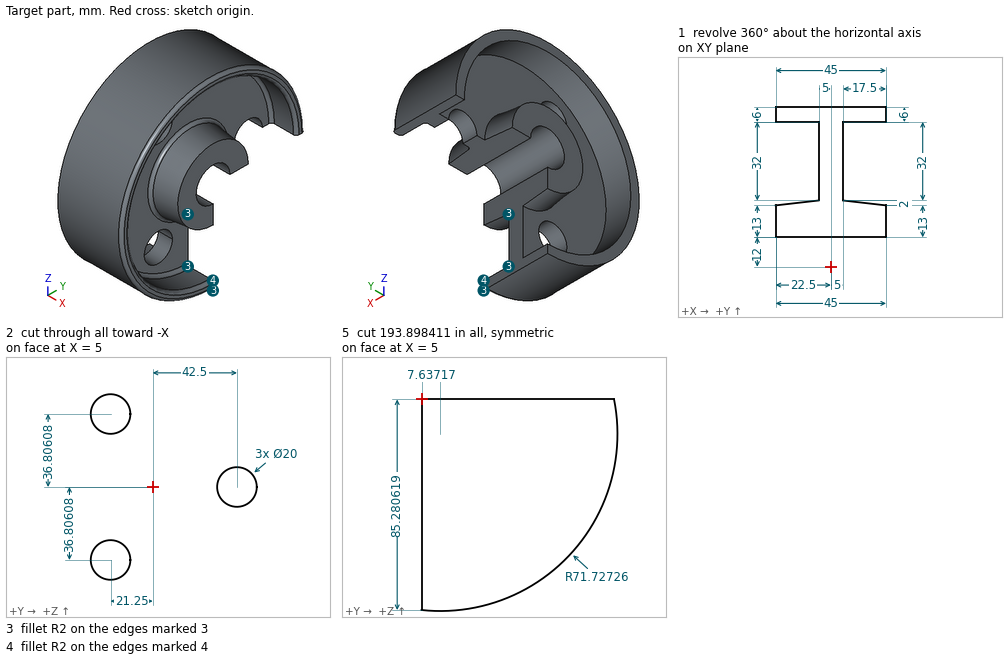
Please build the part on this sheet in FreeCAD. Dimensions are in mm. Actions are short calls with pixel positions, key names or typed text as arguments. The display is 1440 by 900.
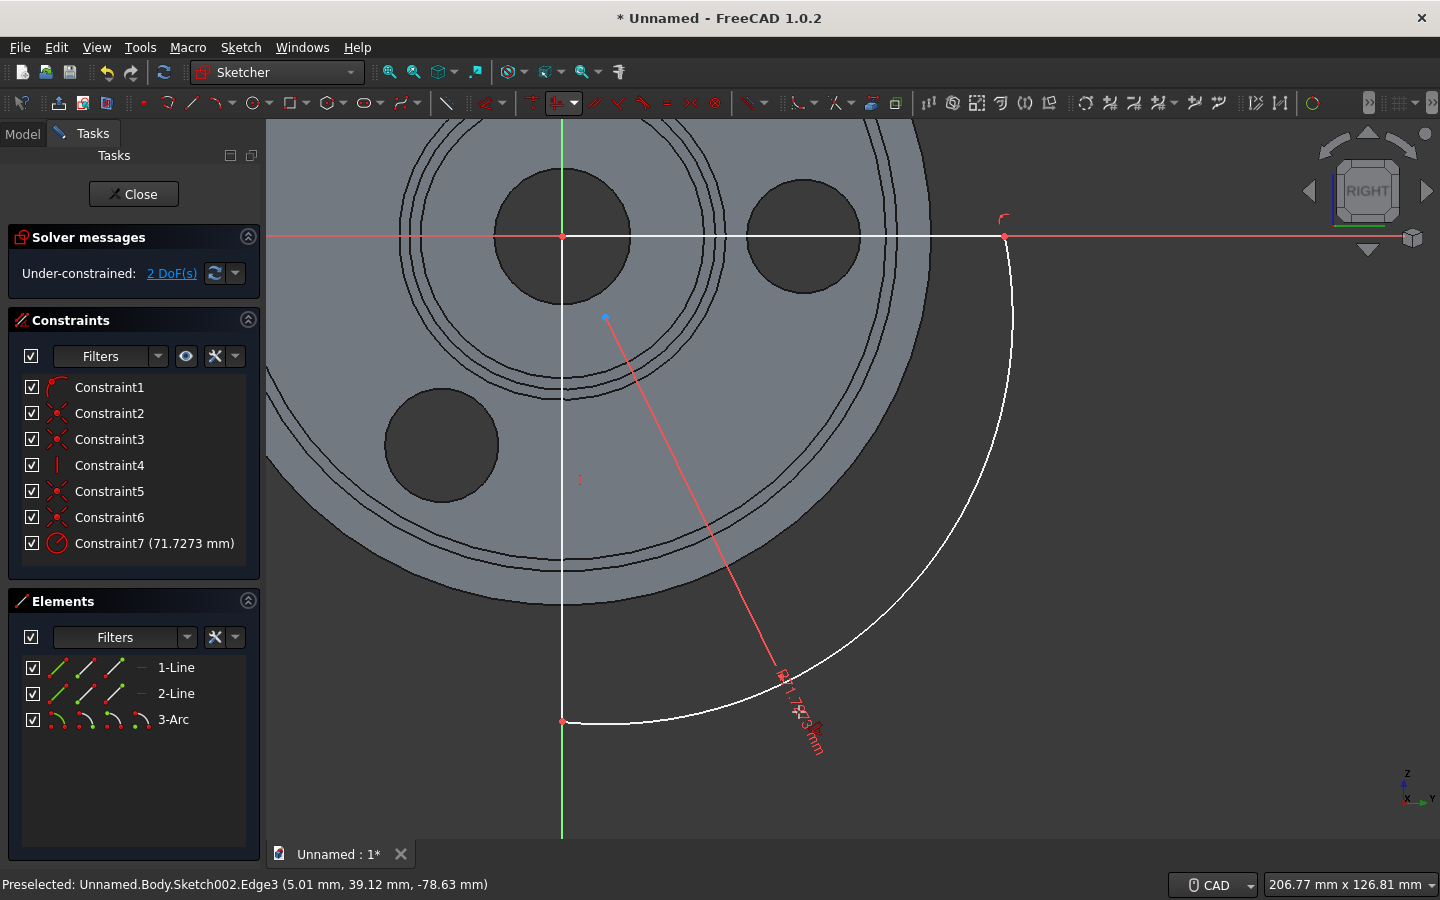
click(605, 317)
click(584, 202)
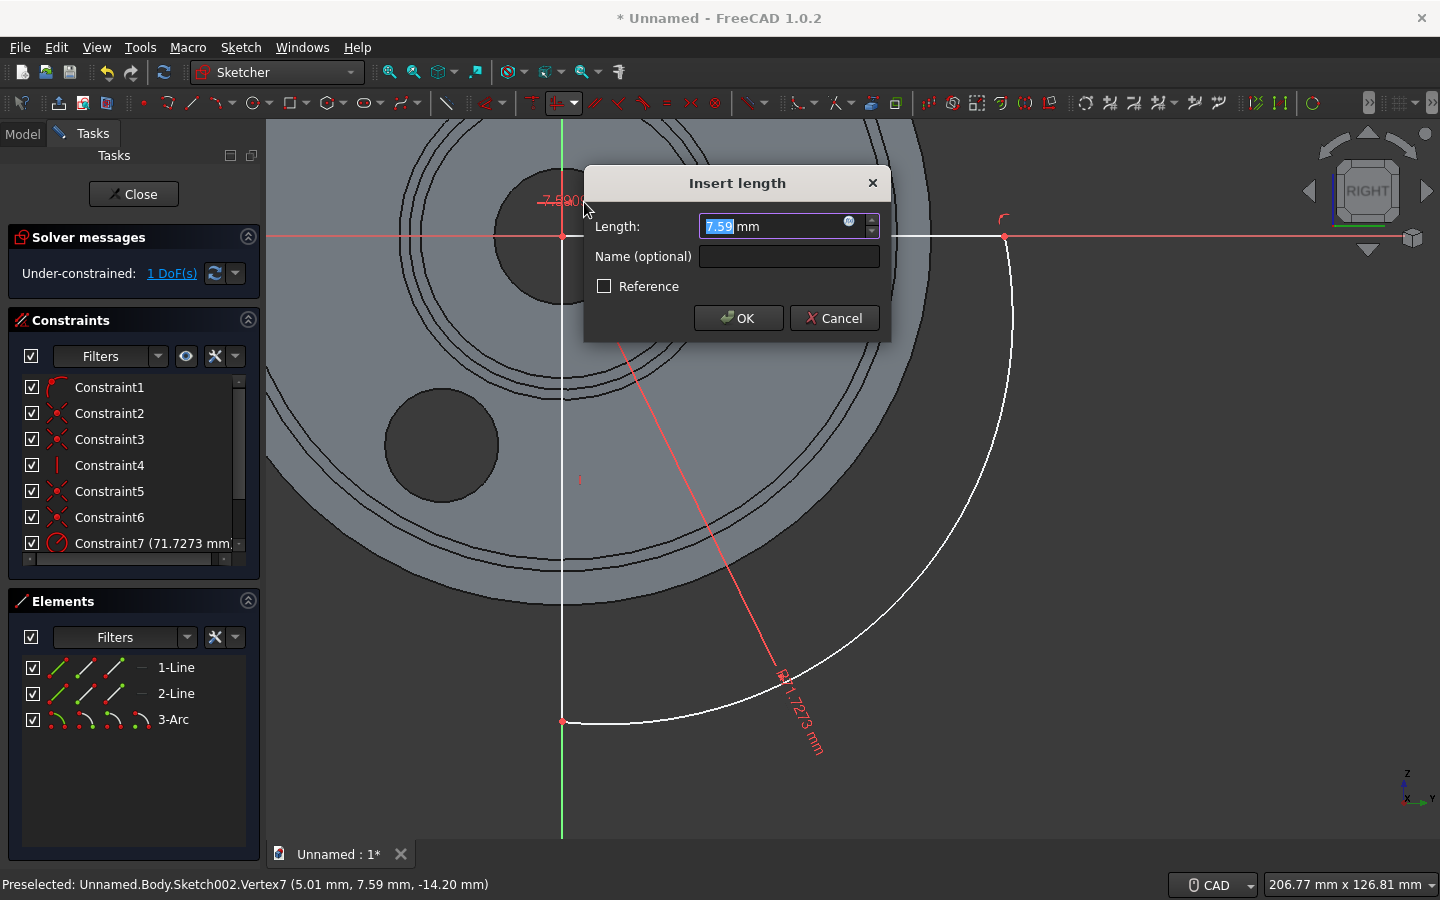
text(7.63717)
key(Return)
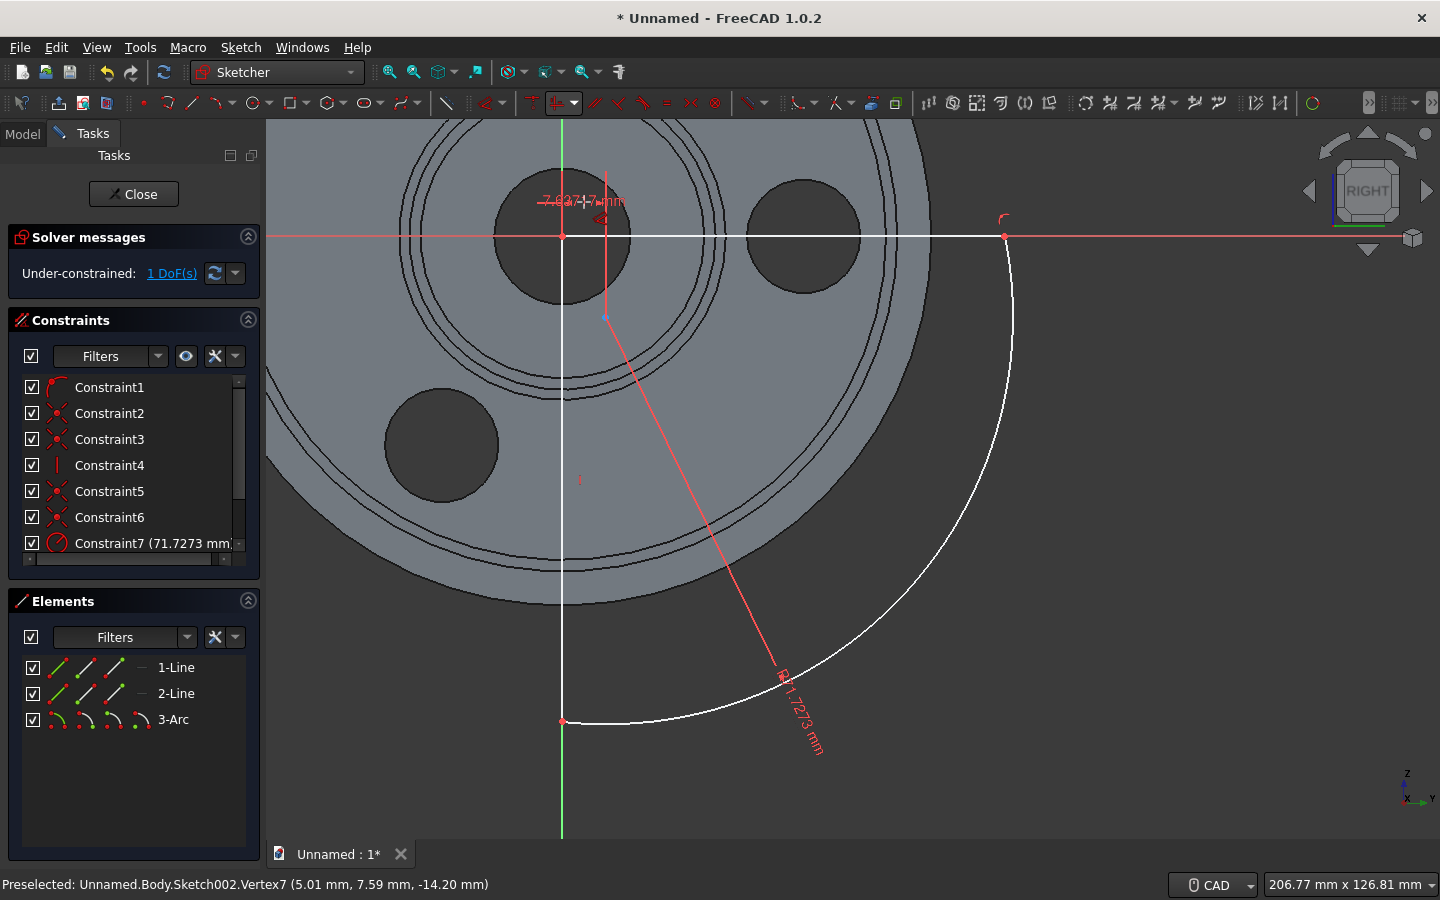
click(562, 382)
click(528, 479)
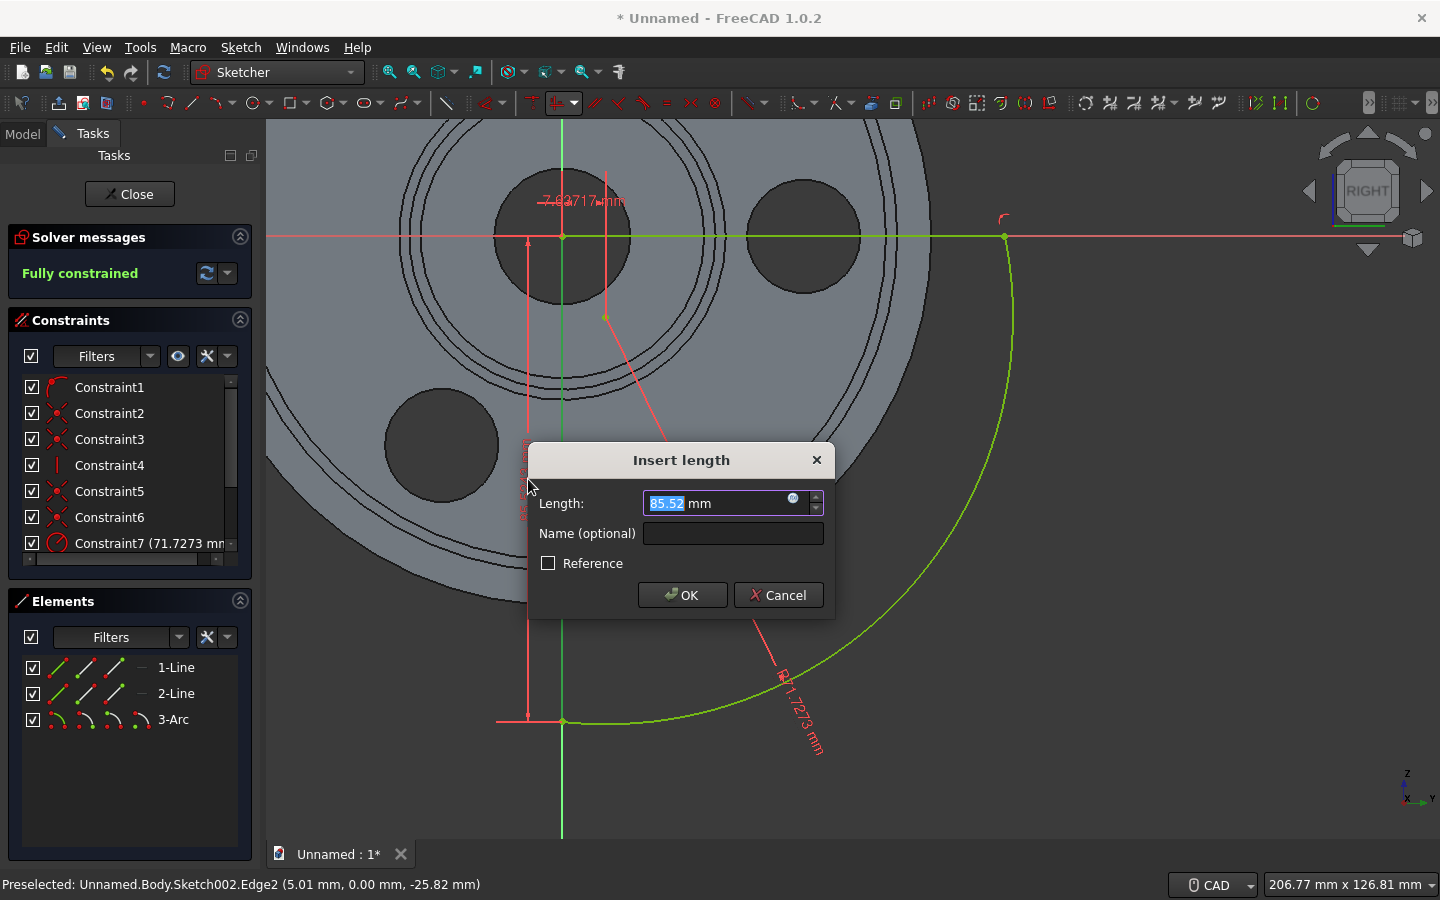
text(85.280619)
key(Return)
key(Escape)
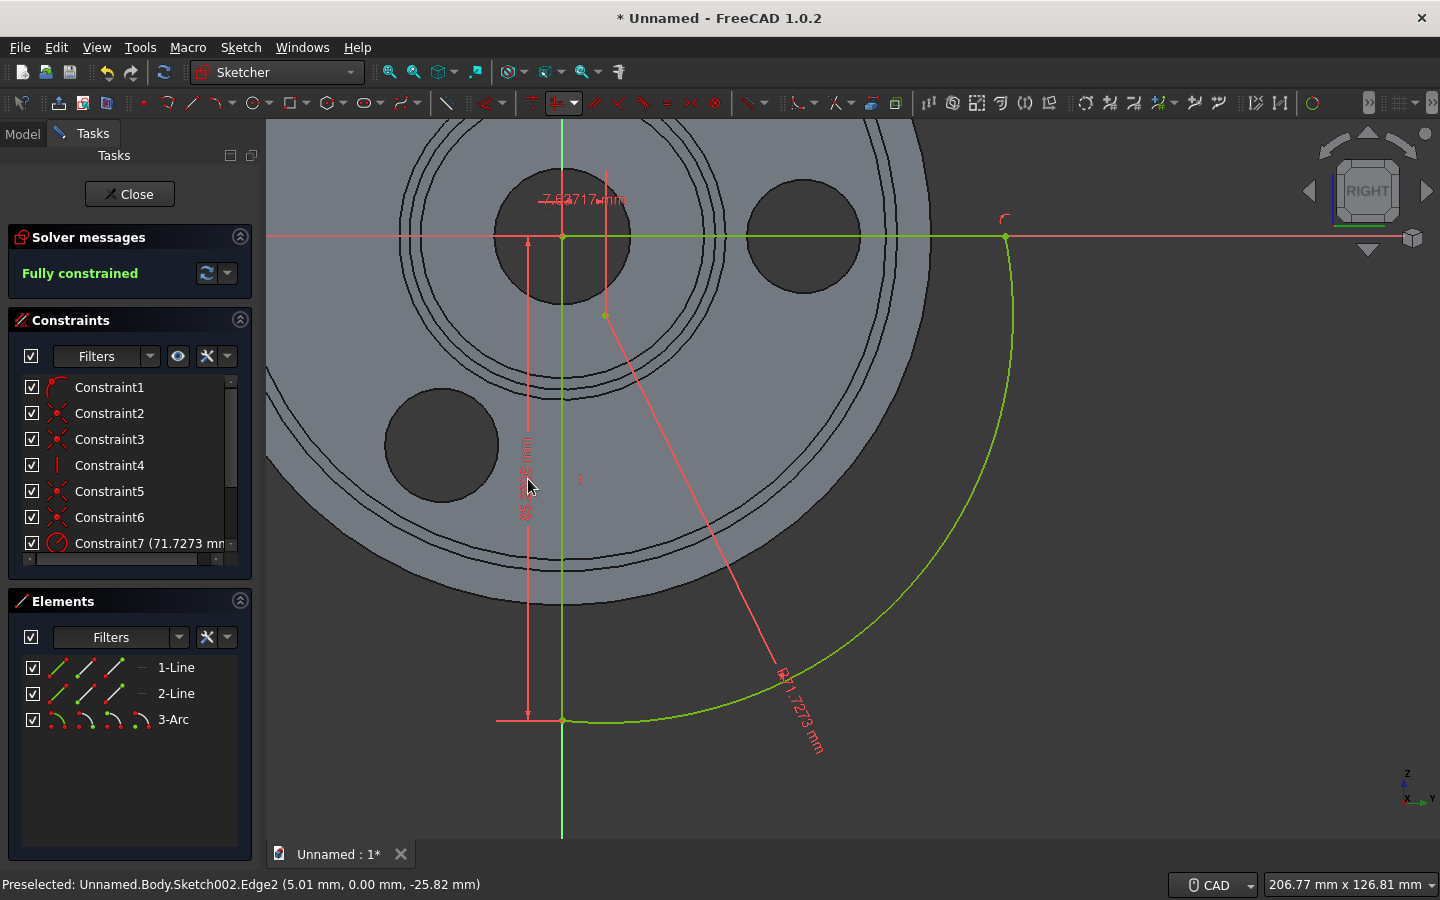
click(130, 194)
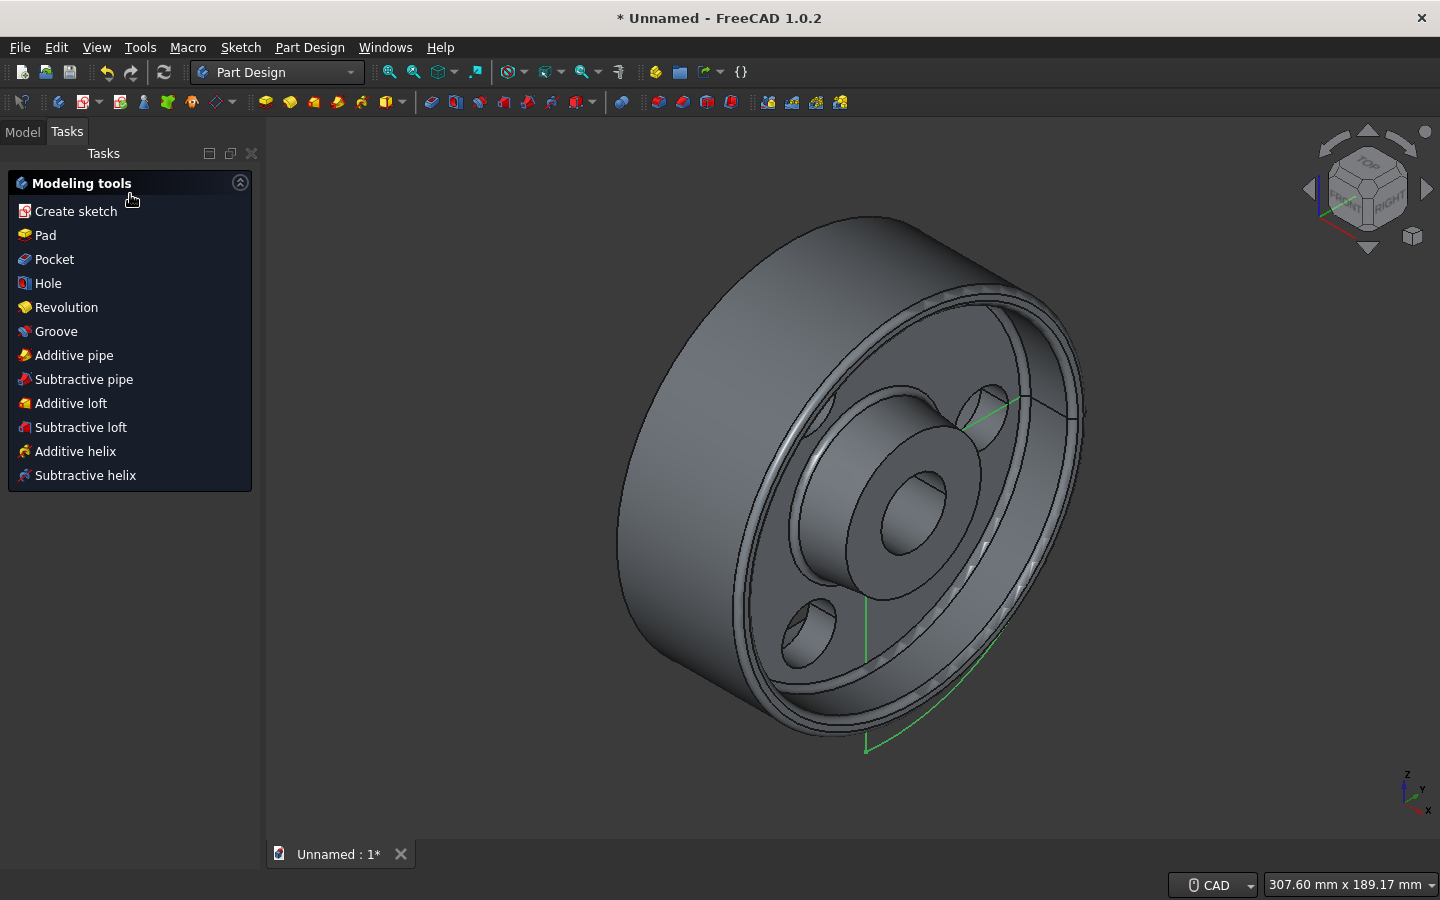
click(432, 102)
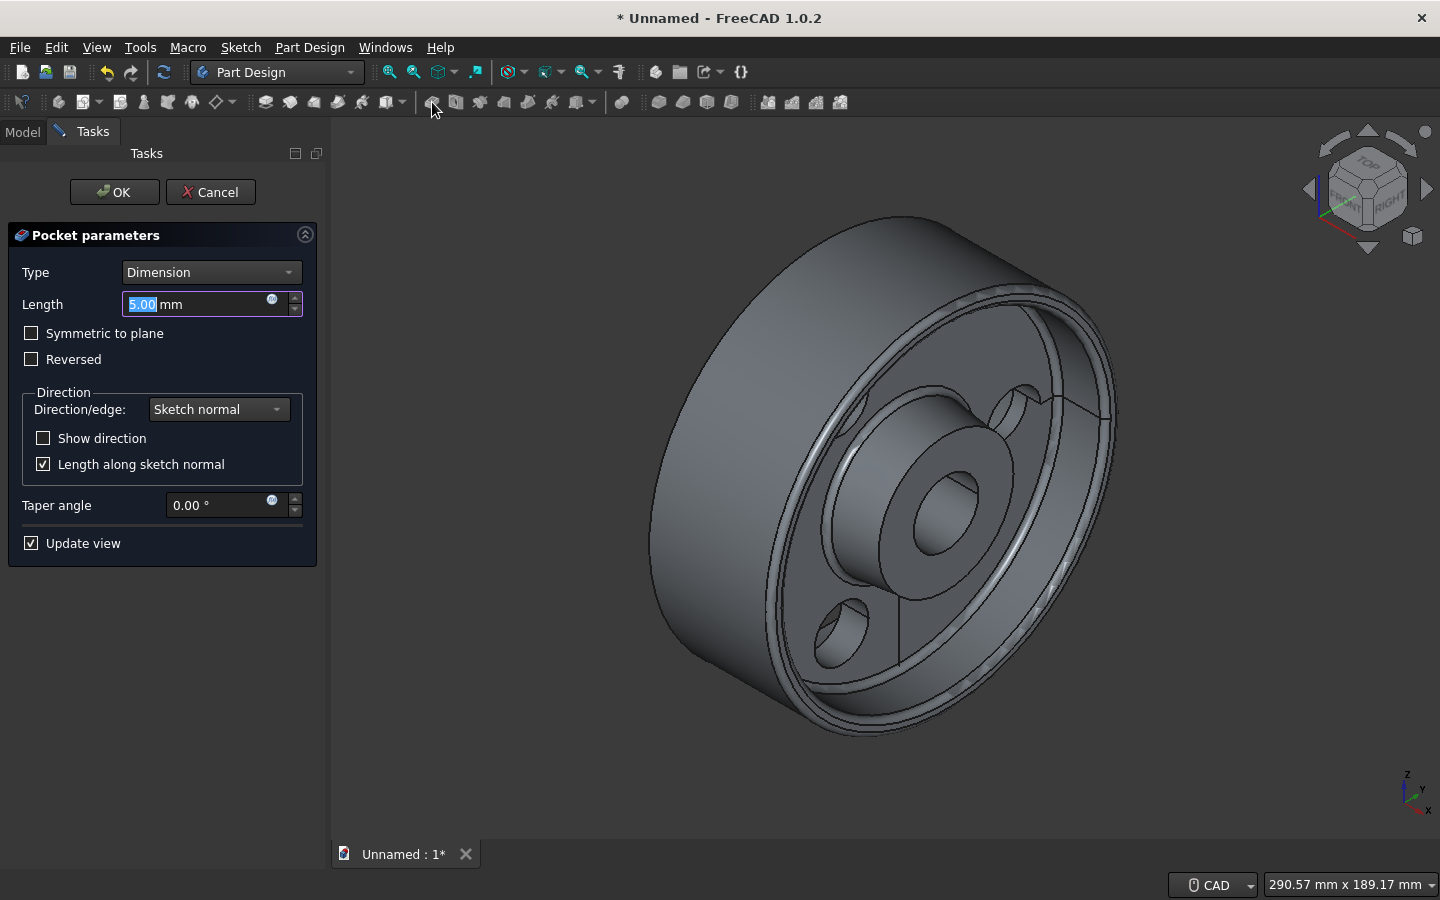
text(193.898411)
key(Tab)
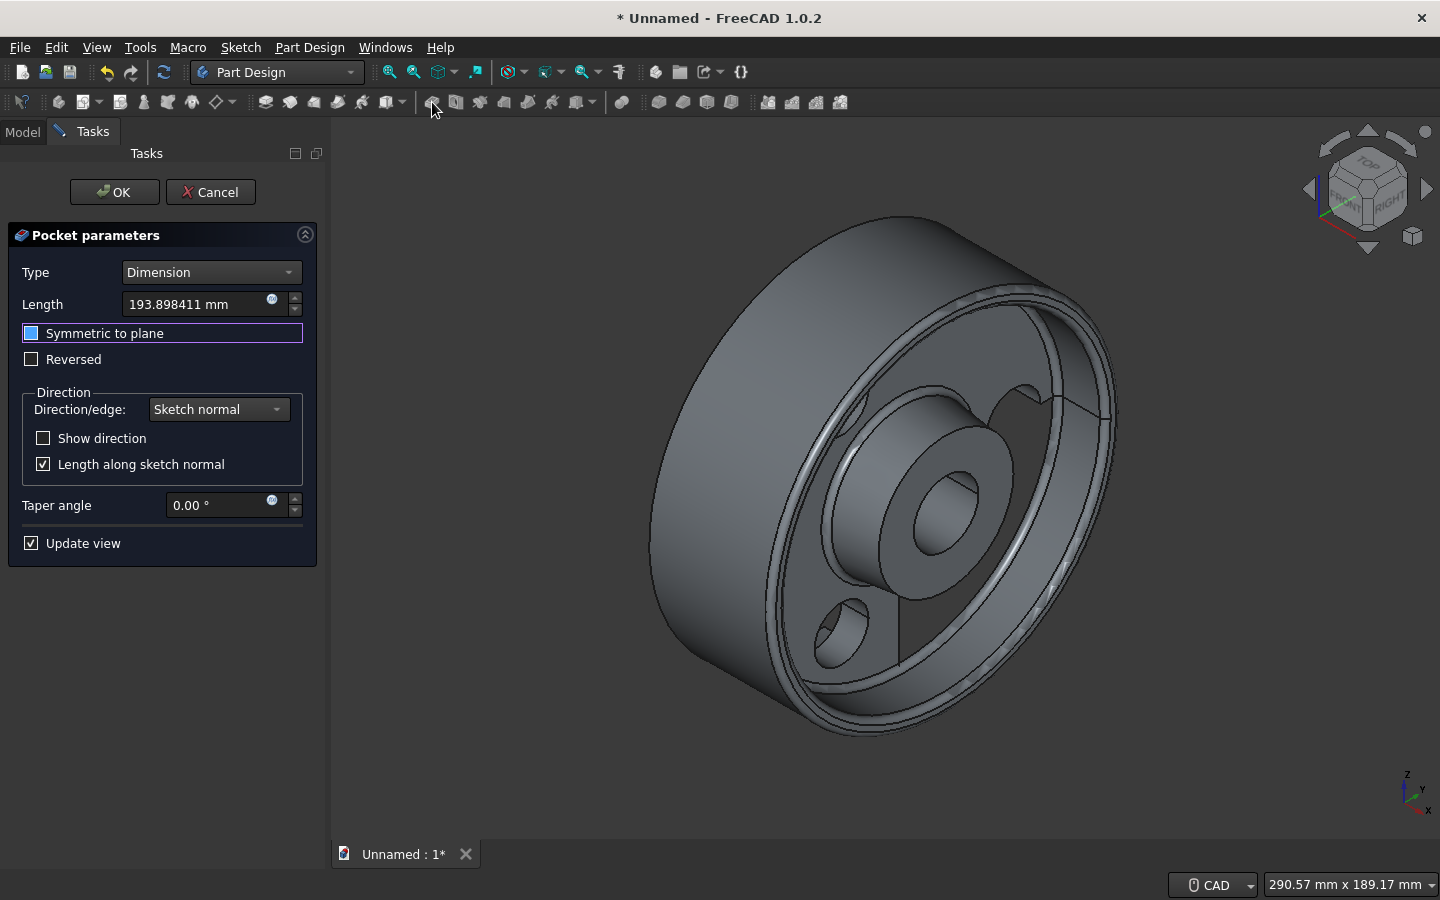
click(30, 333)